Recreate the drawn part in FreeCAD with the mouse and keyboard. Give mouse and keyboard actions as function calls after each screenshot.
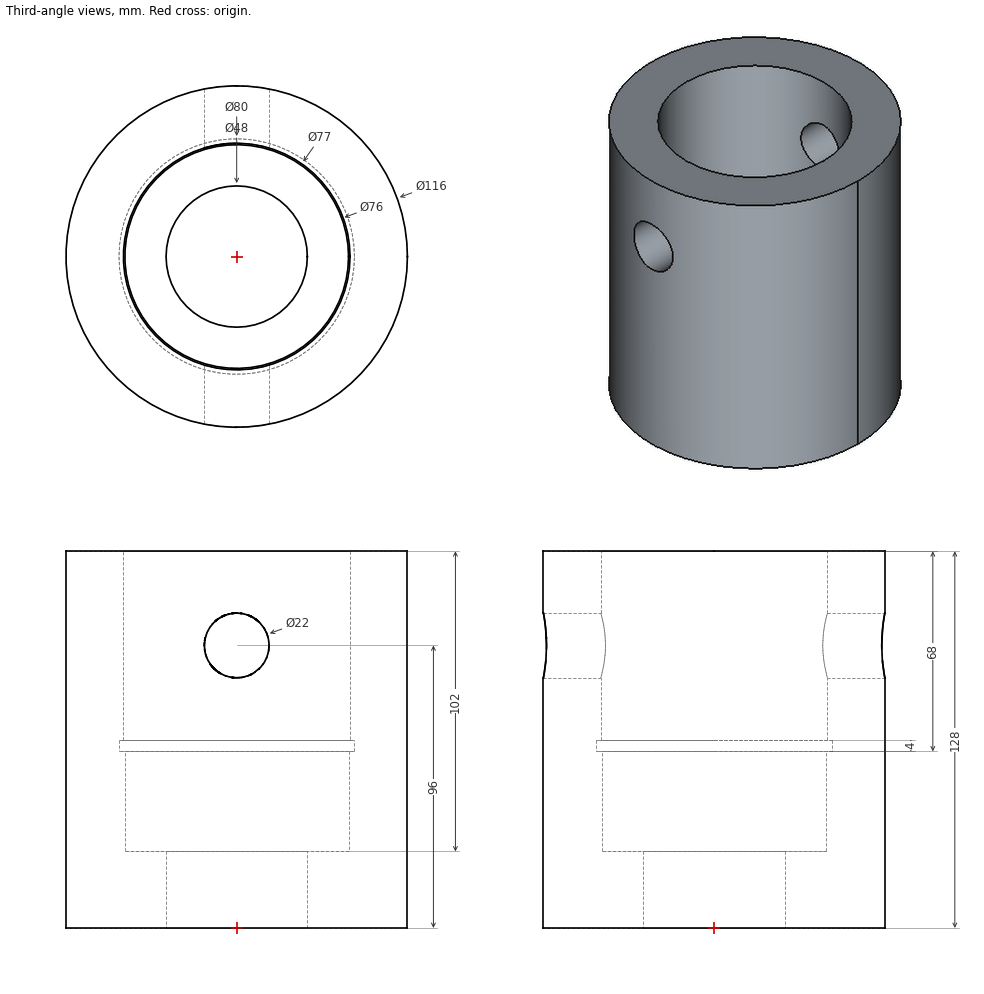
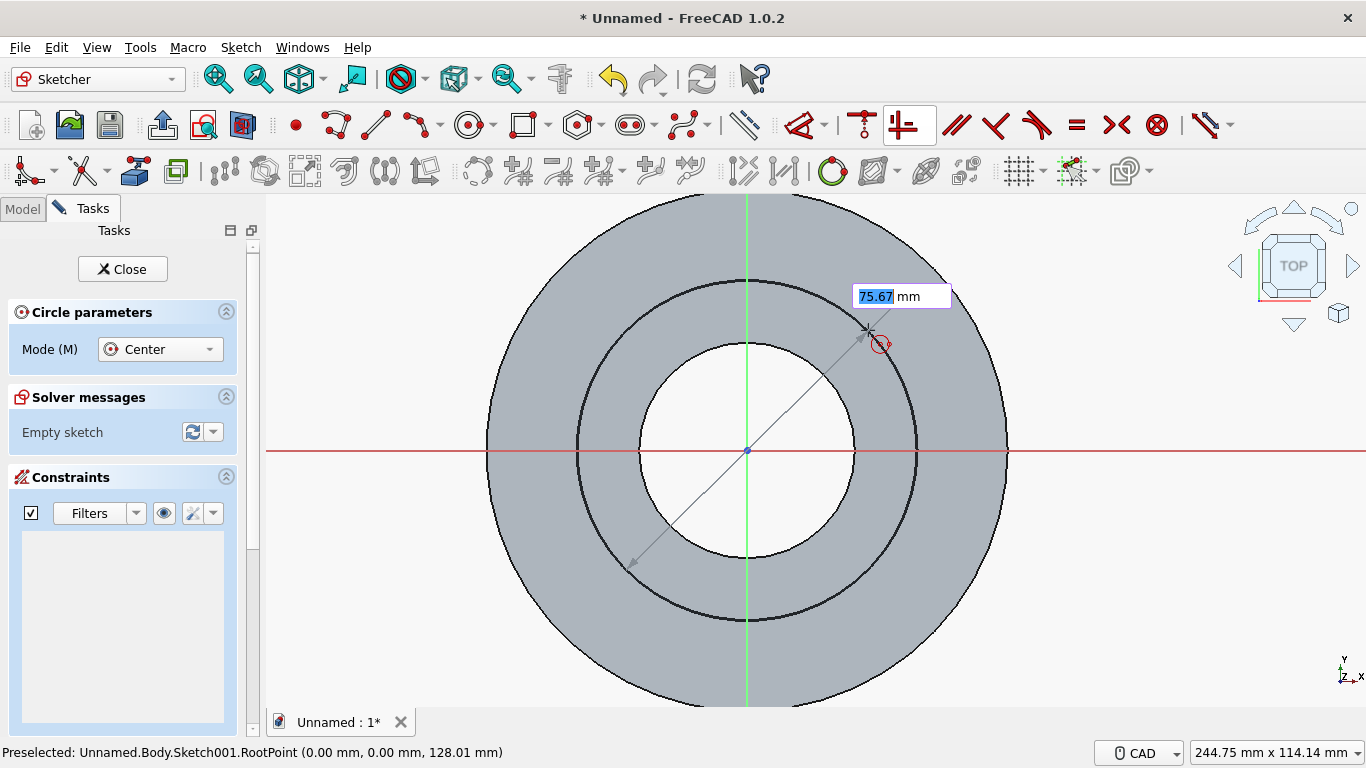
text(76)
key(Return)
key(Escape)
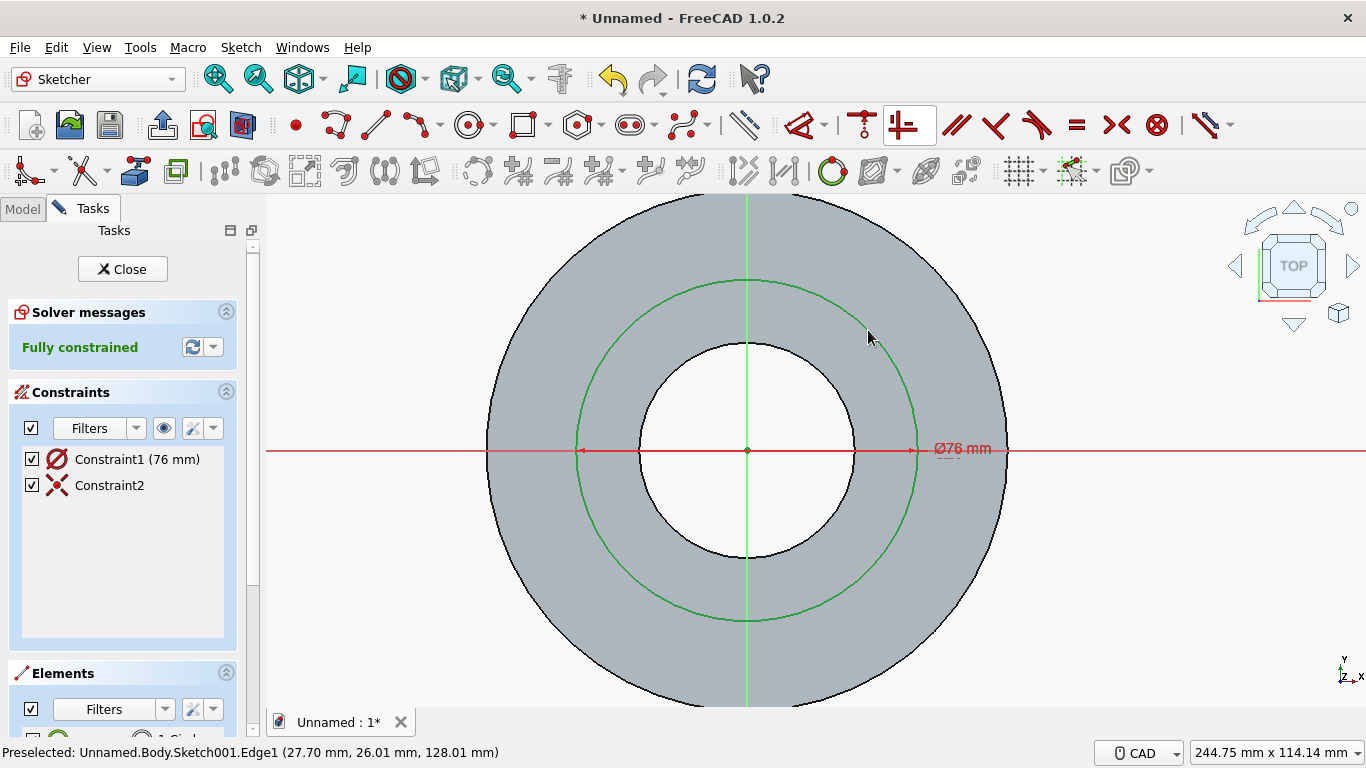
click(123, 269)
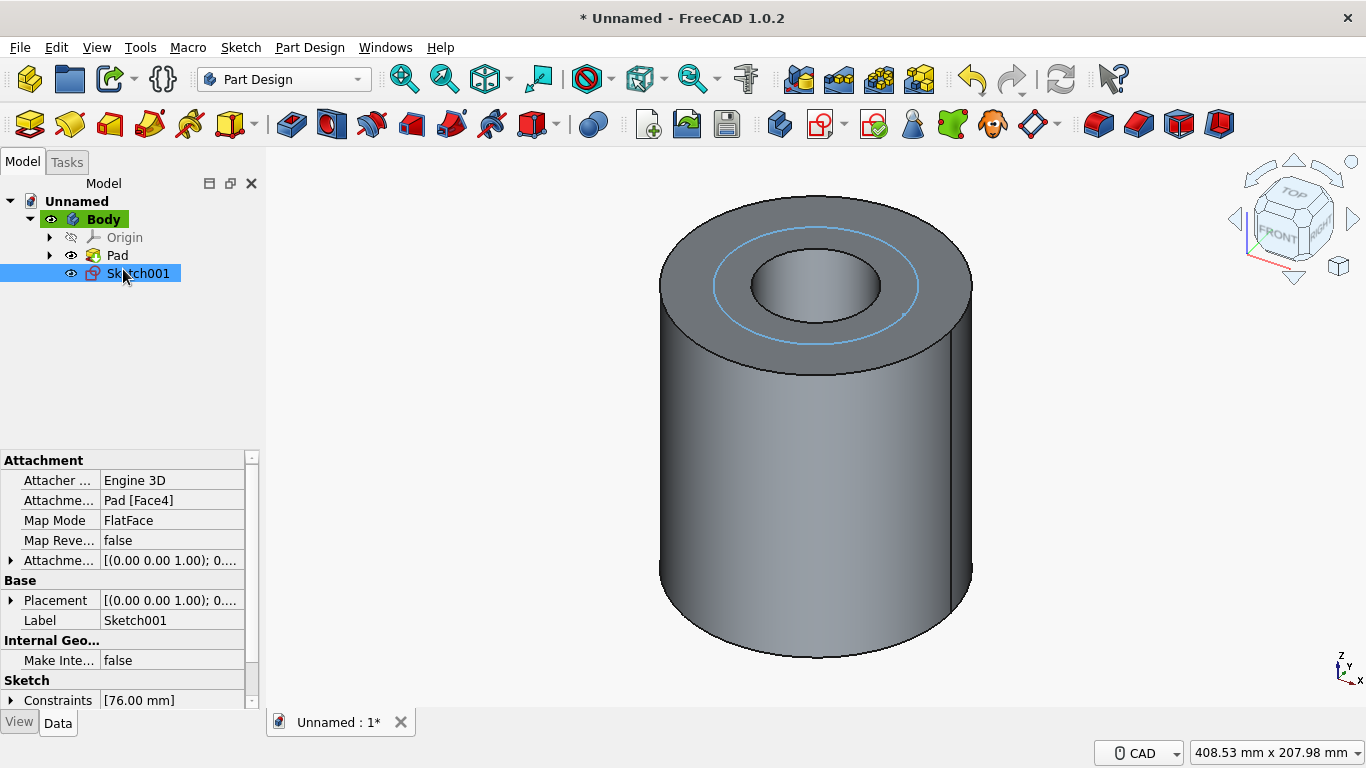
click(292, 124)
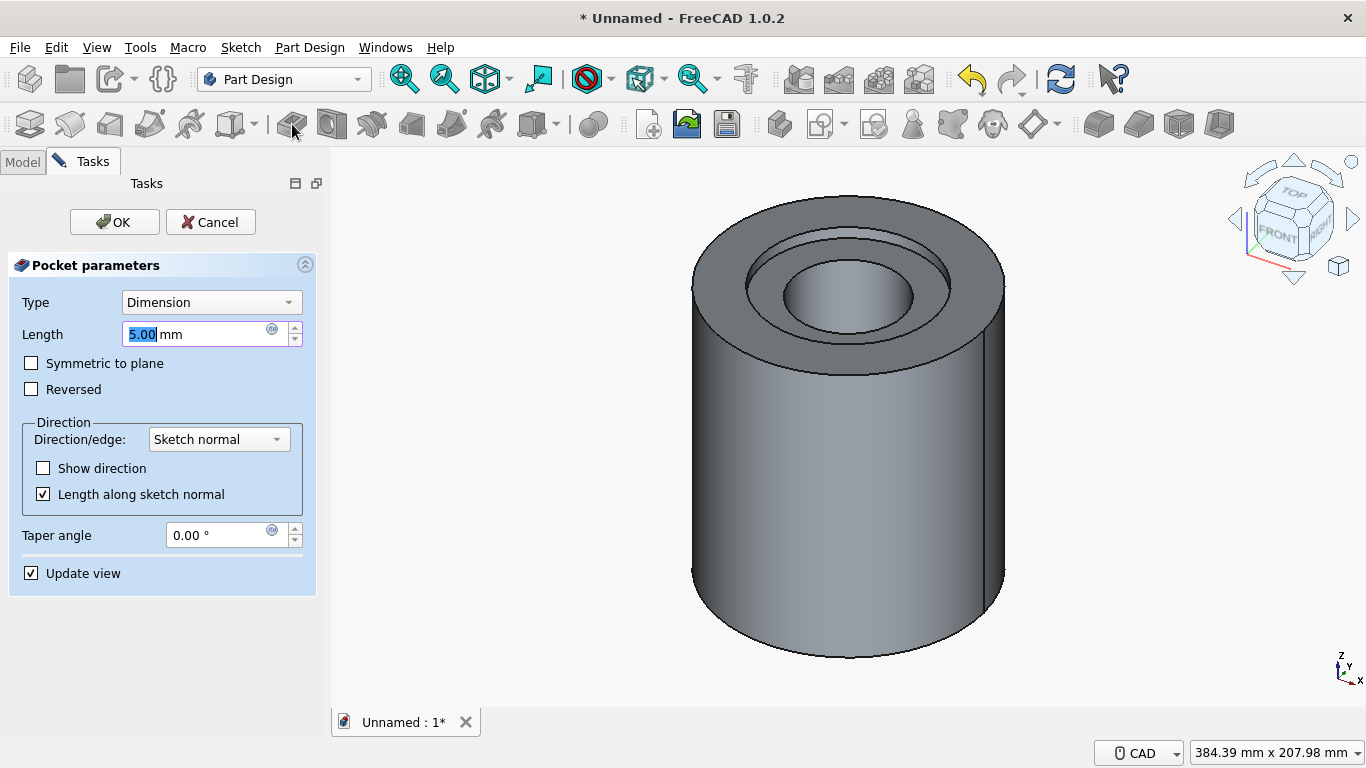
text(102)
key(Tab)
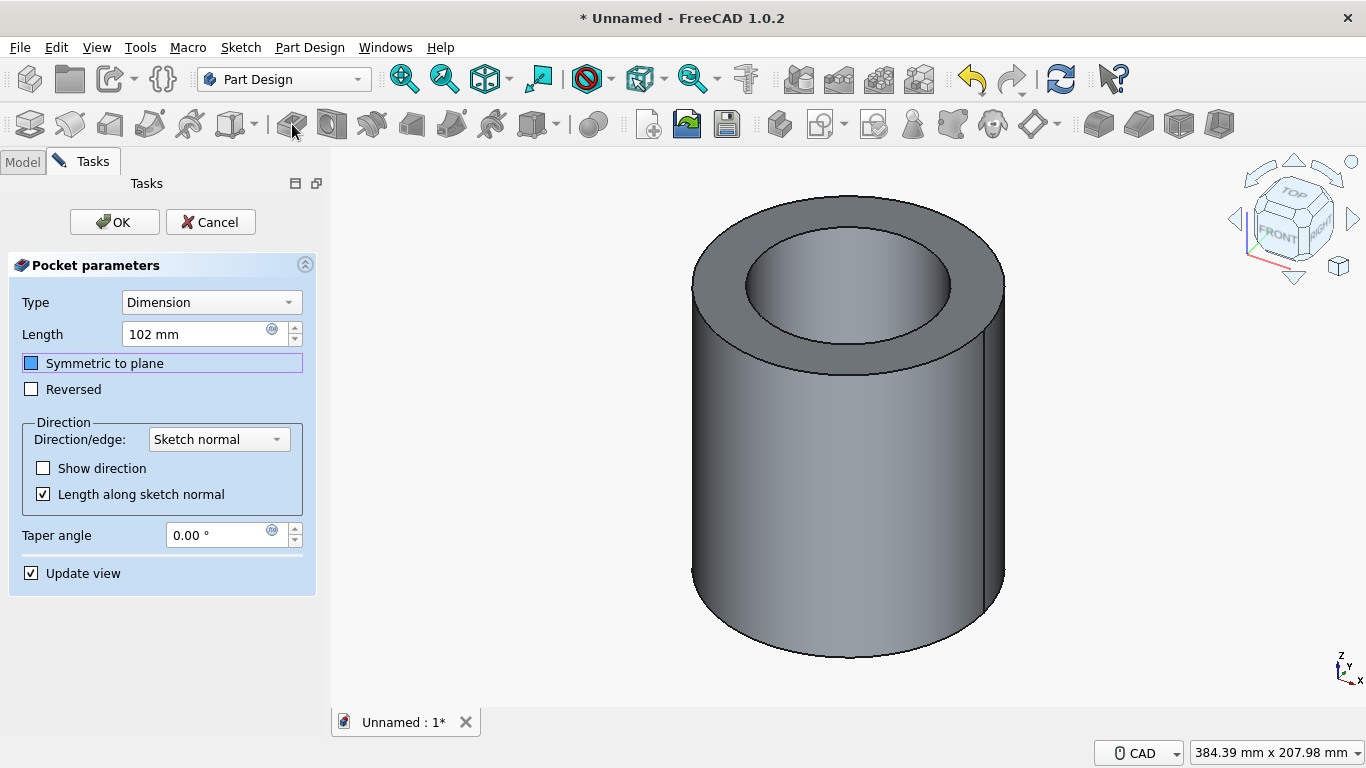
click(115, 222)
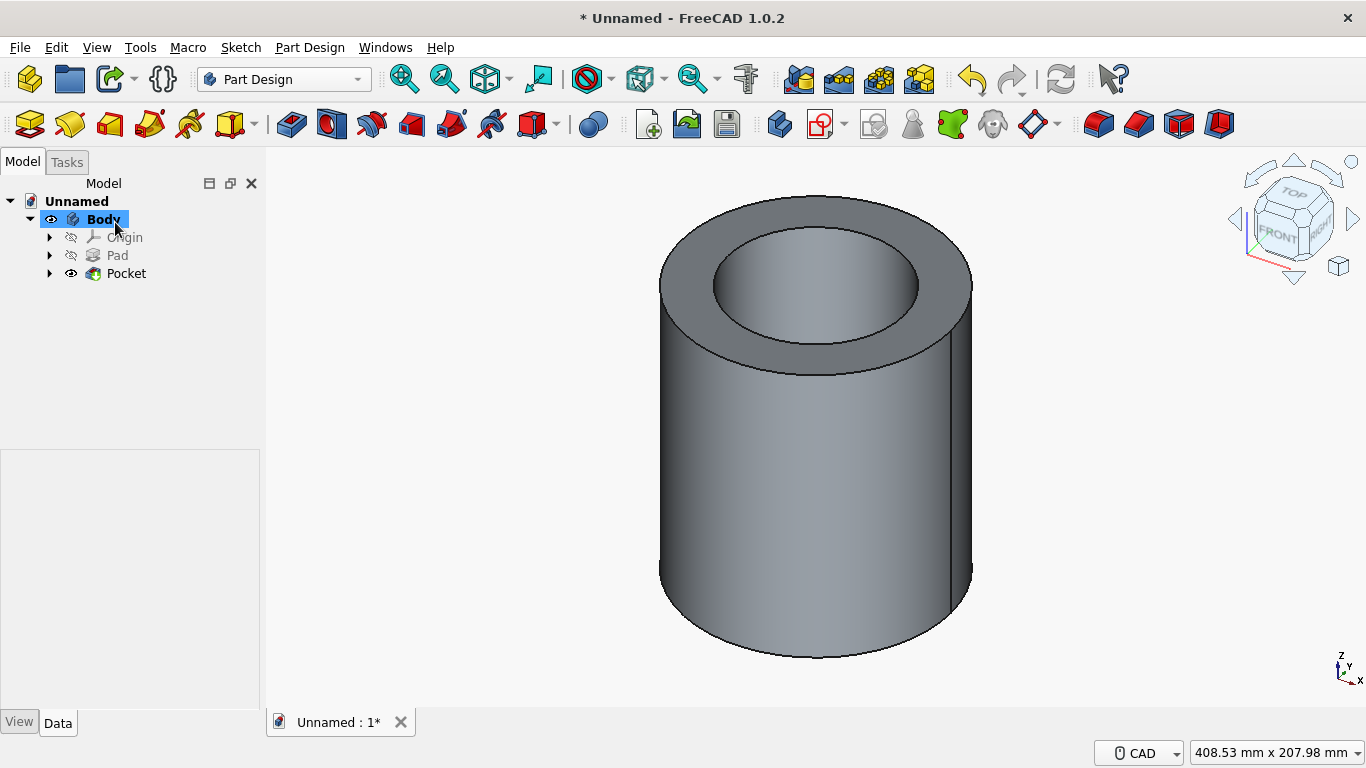
click(820, 124)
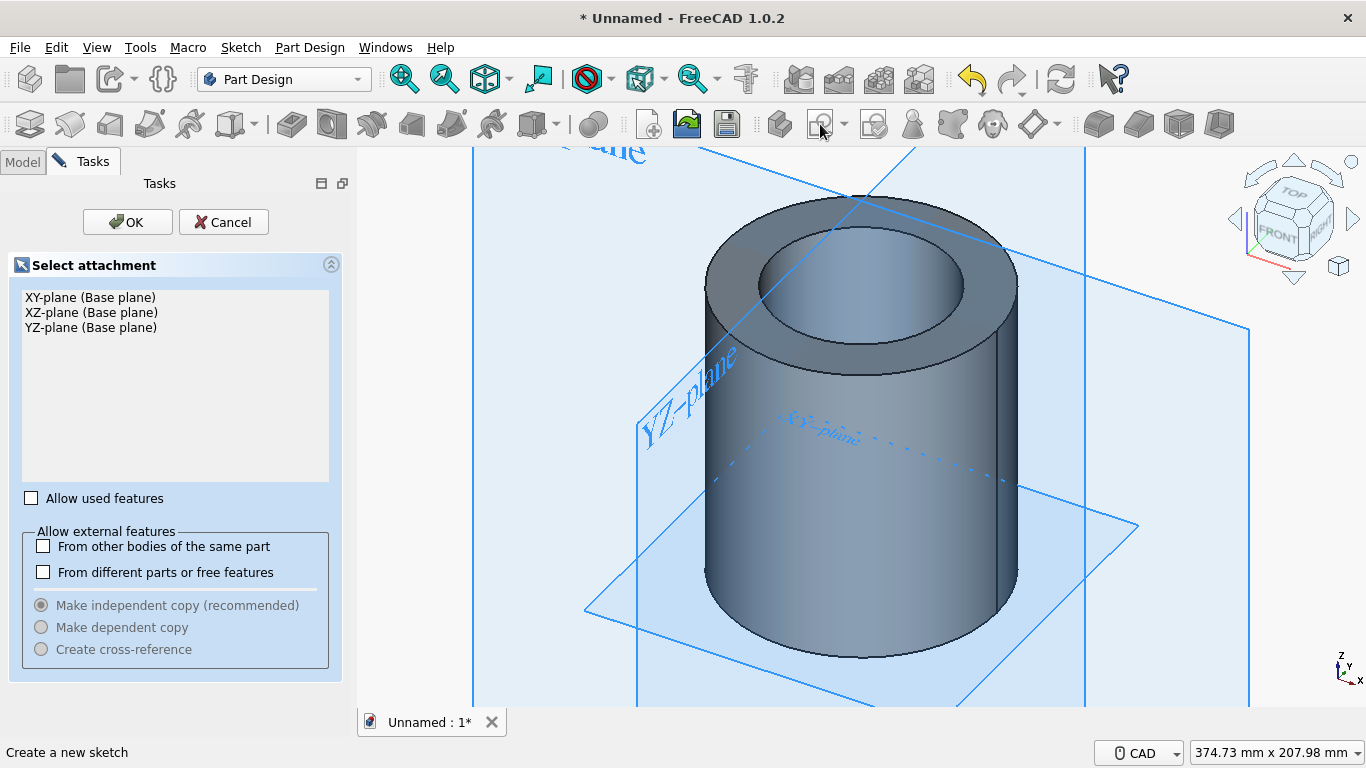
click(82, 312)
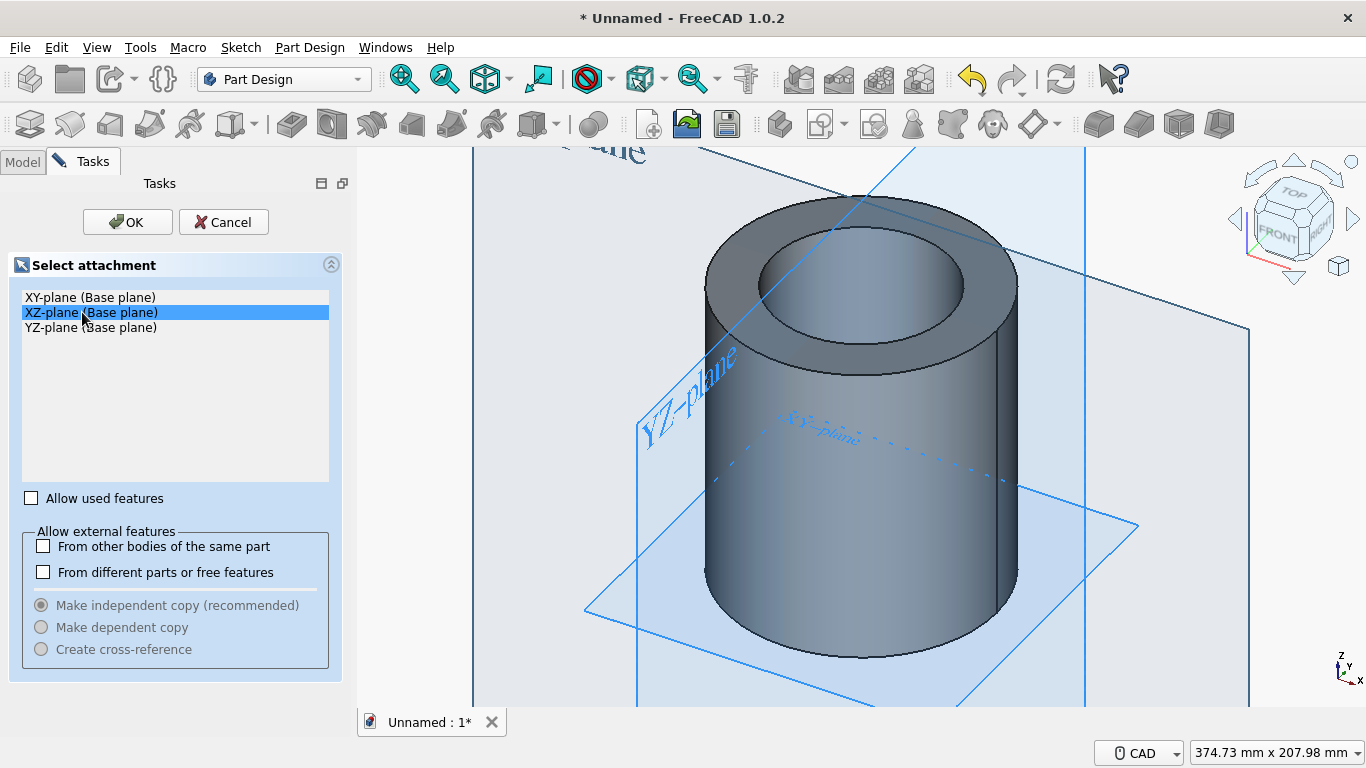
click(128, 222)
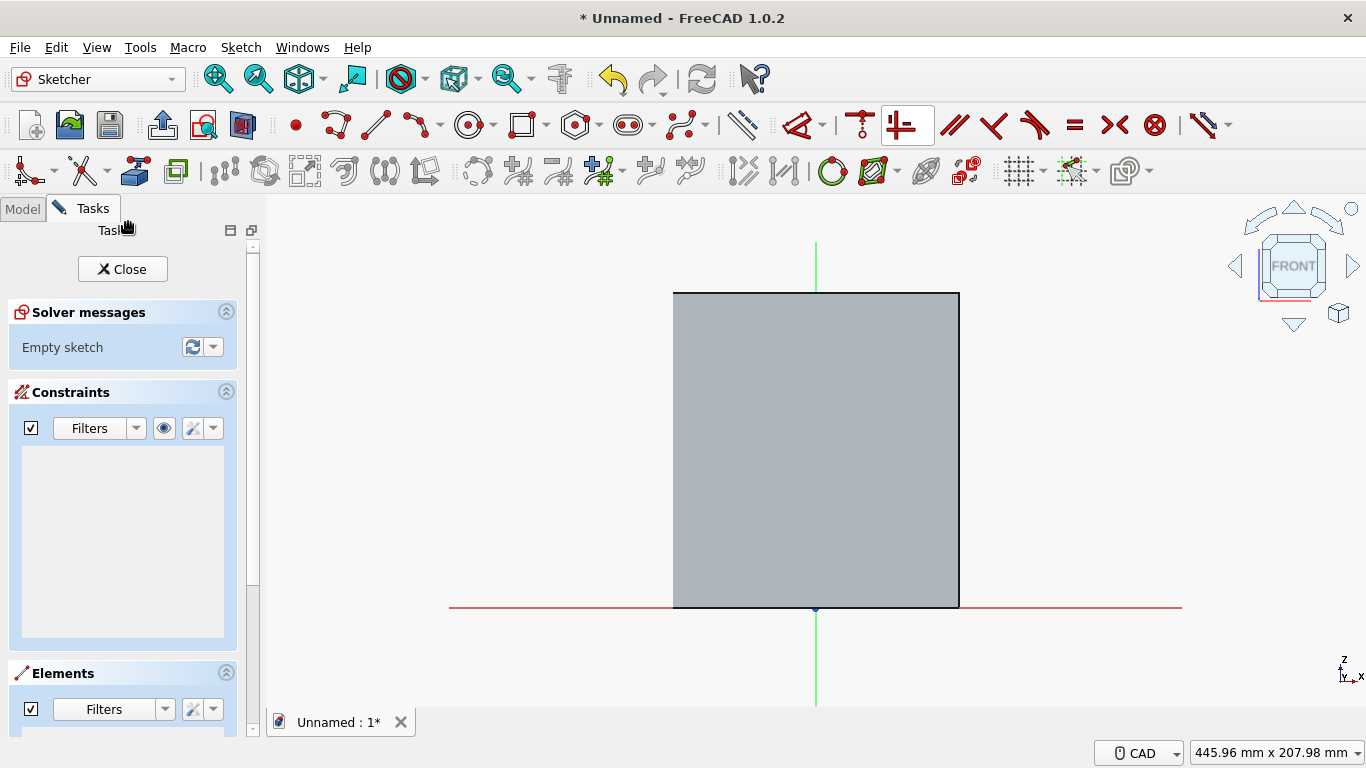
click(244, 126)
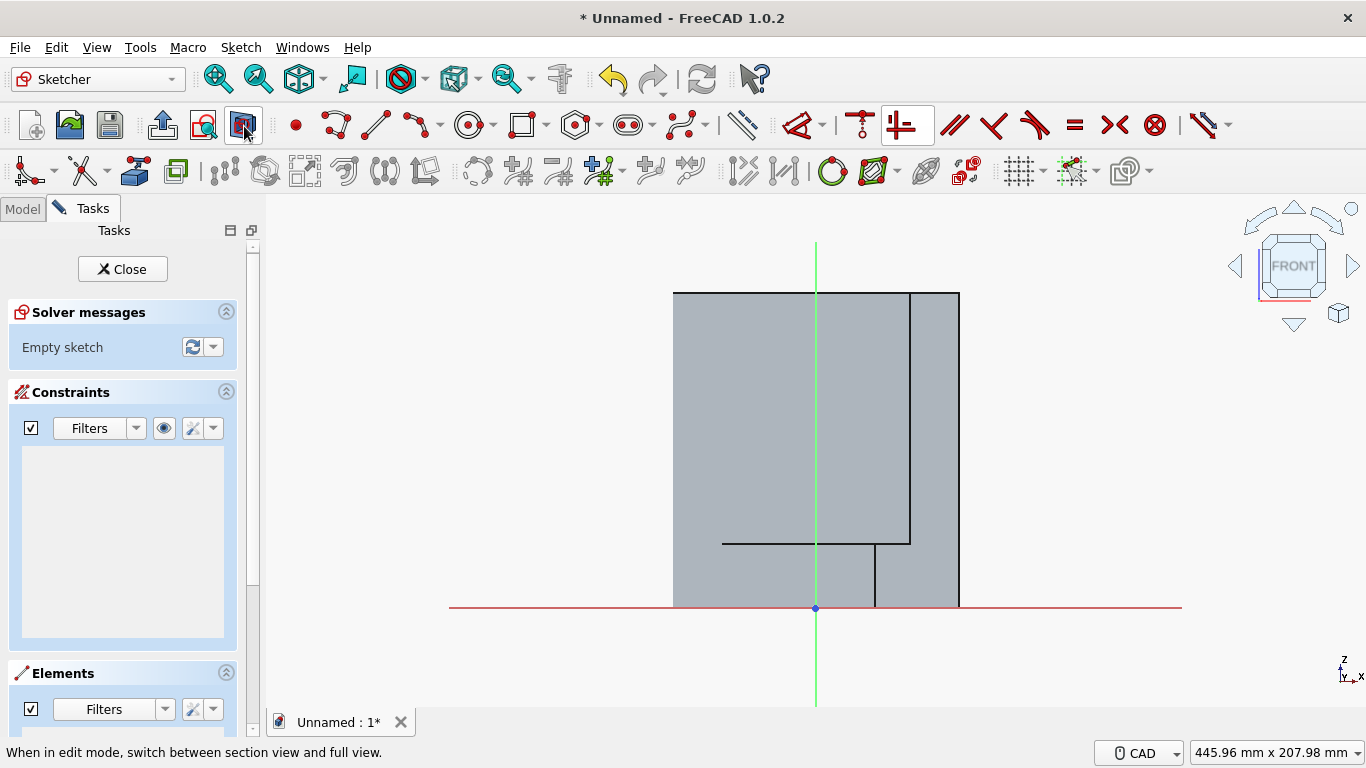
scroll(829, 356, up, 9)